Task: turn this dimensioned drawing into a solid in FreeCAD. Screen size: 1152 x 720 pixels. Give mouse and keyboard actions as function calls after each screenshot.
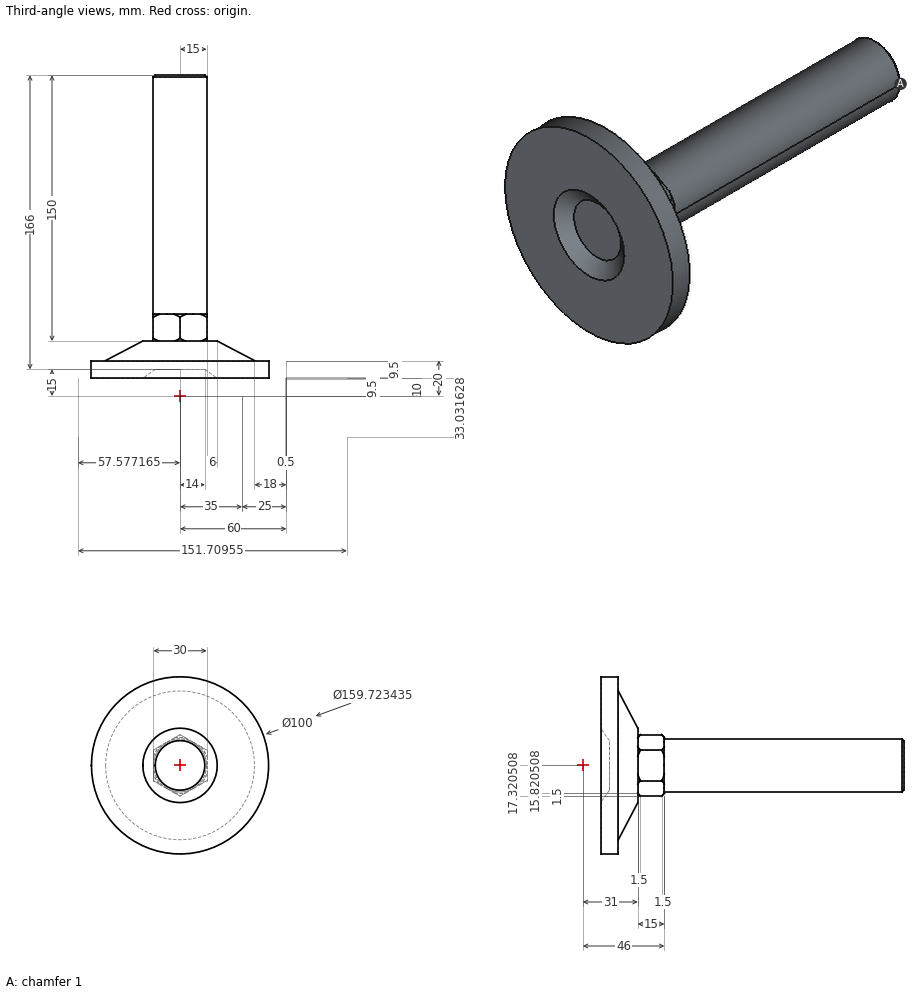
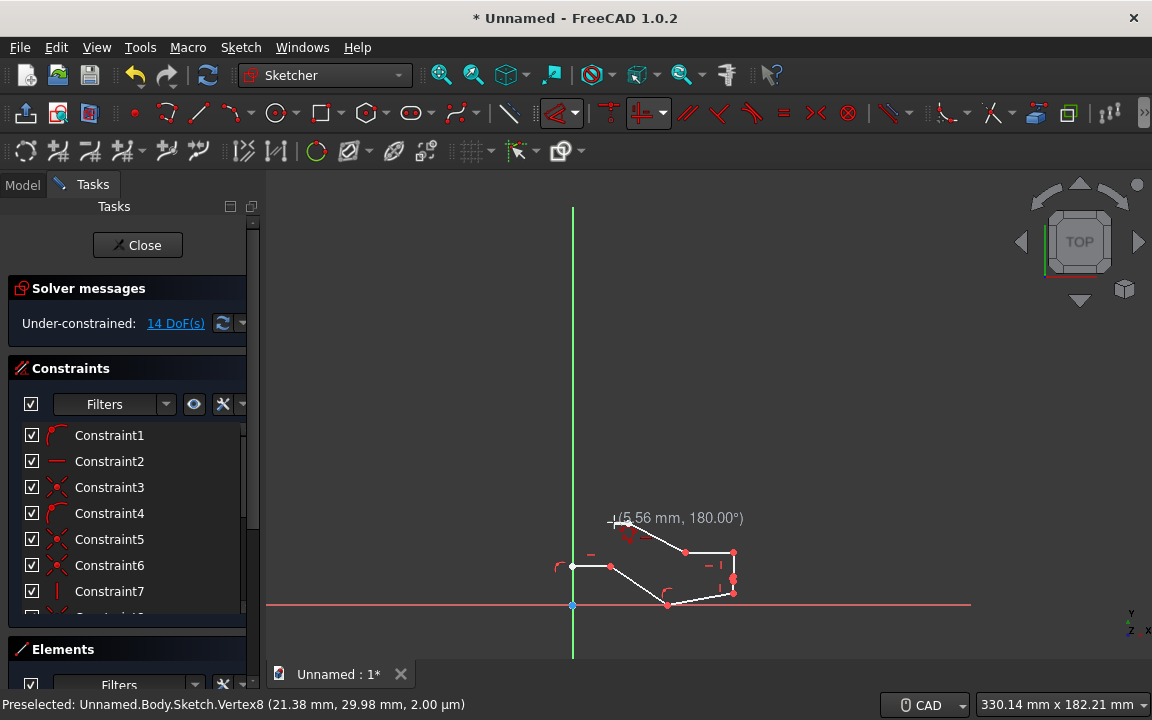
click(613, 522)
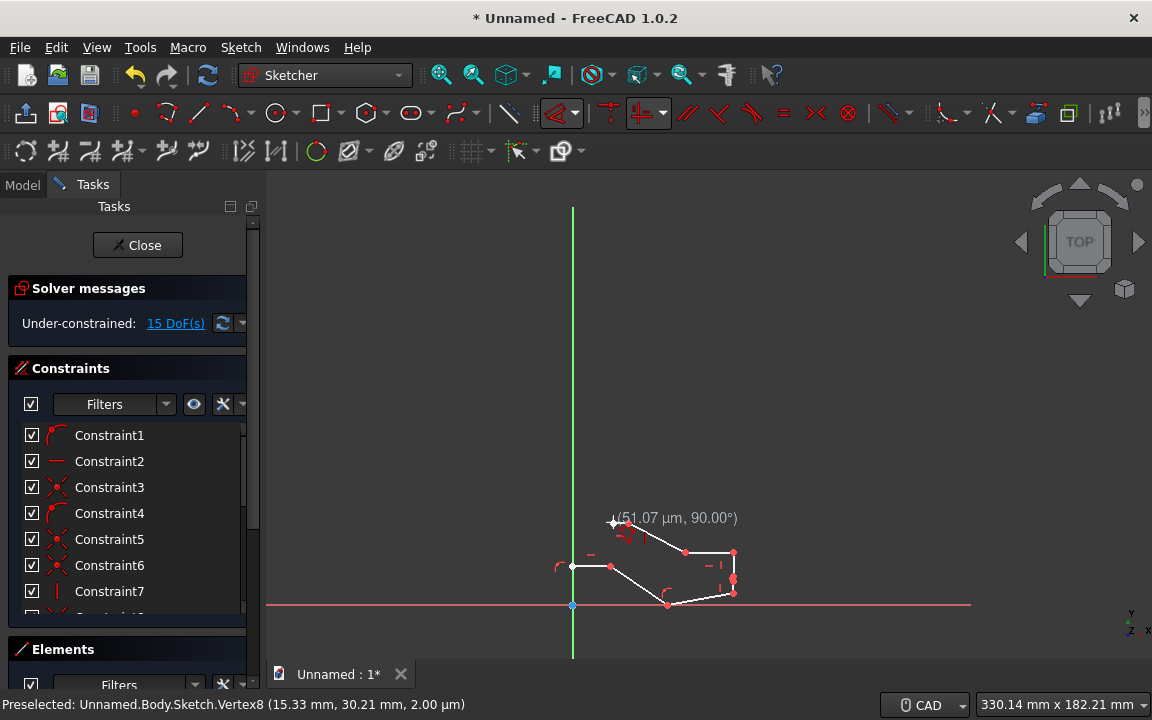
scroll(614, 521, down, 2)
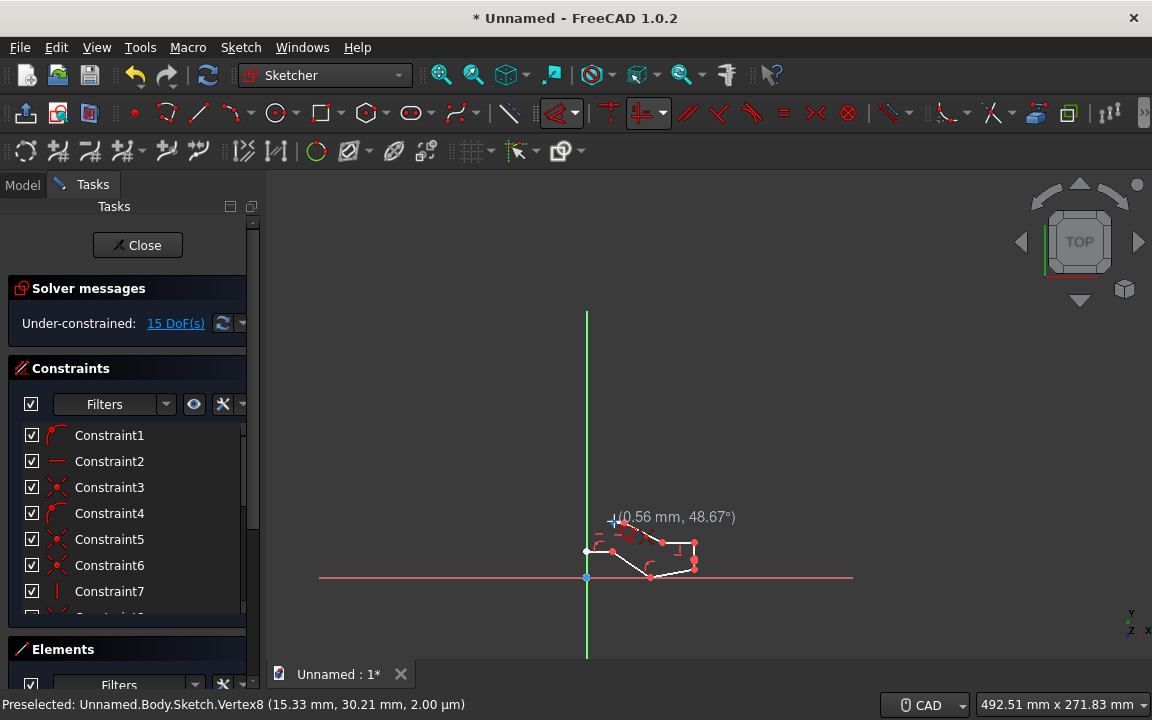
click(613, 252)
click(596, 252)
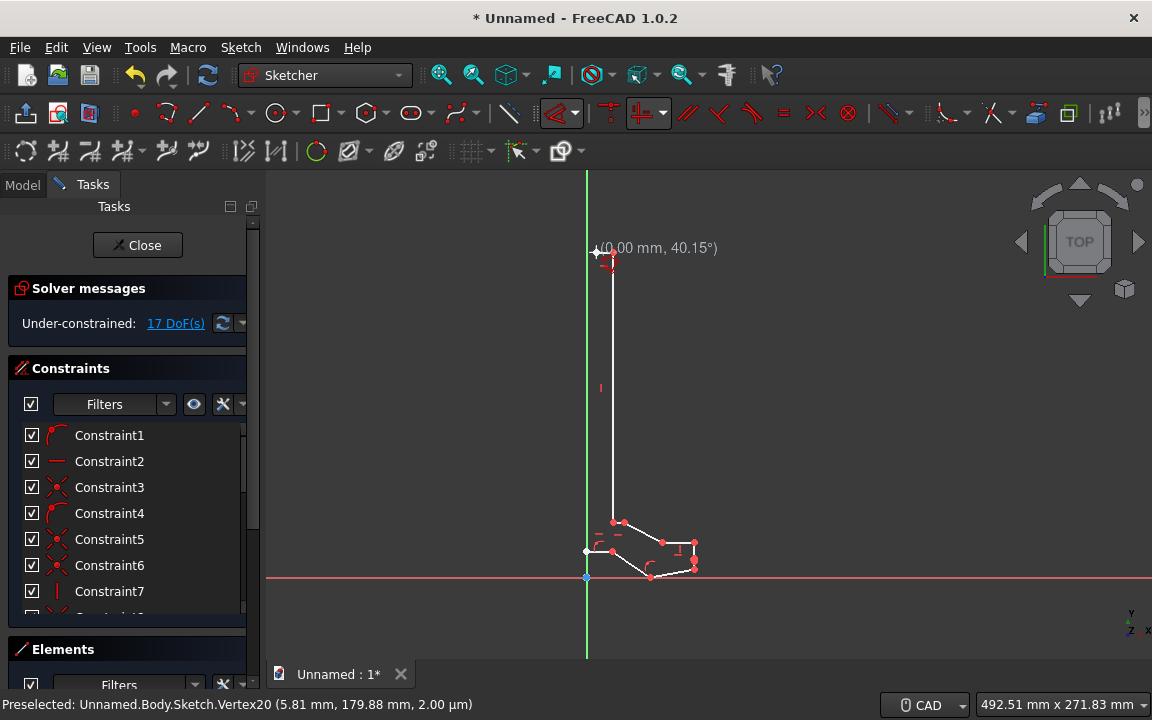
scroll(587, 551, up, 2)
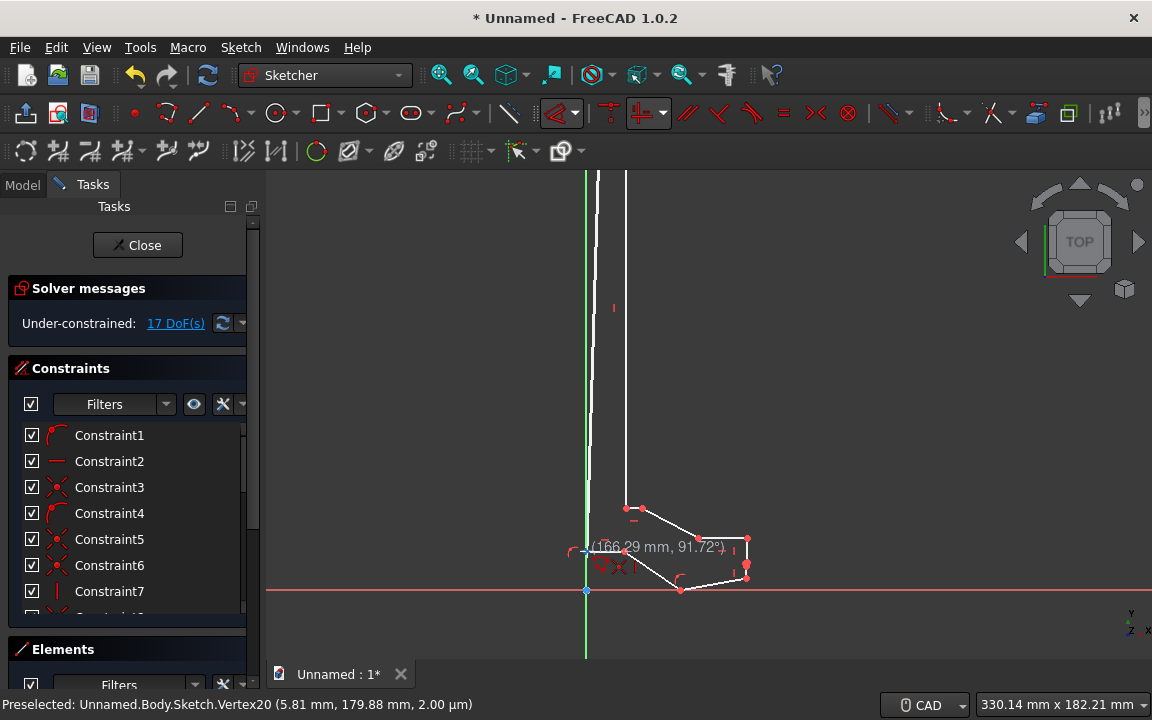
click(586, 552)
key(Escape)
key(Escape)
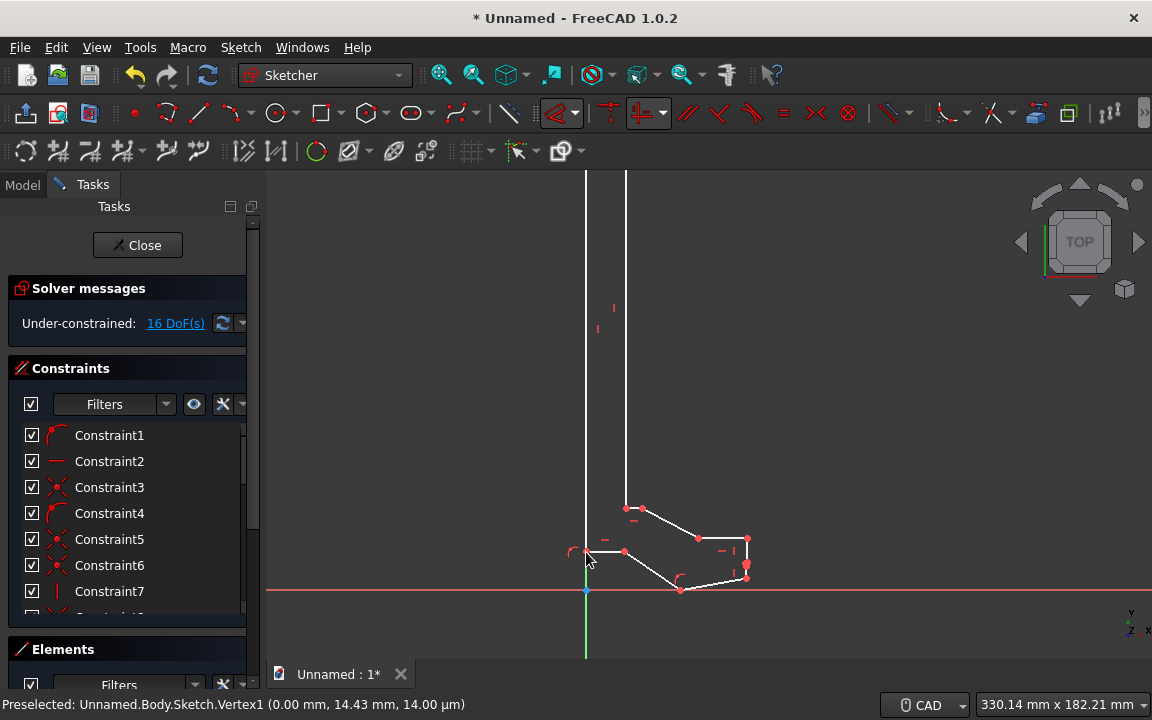
click(700, 587)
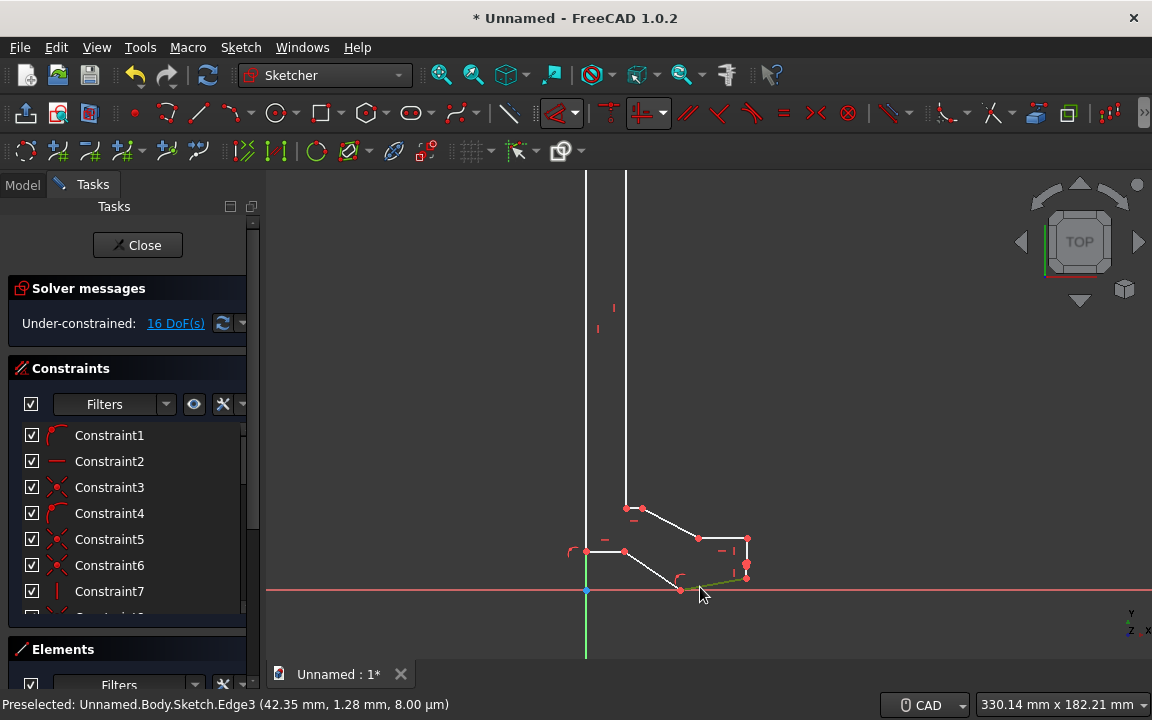
click(666, 114)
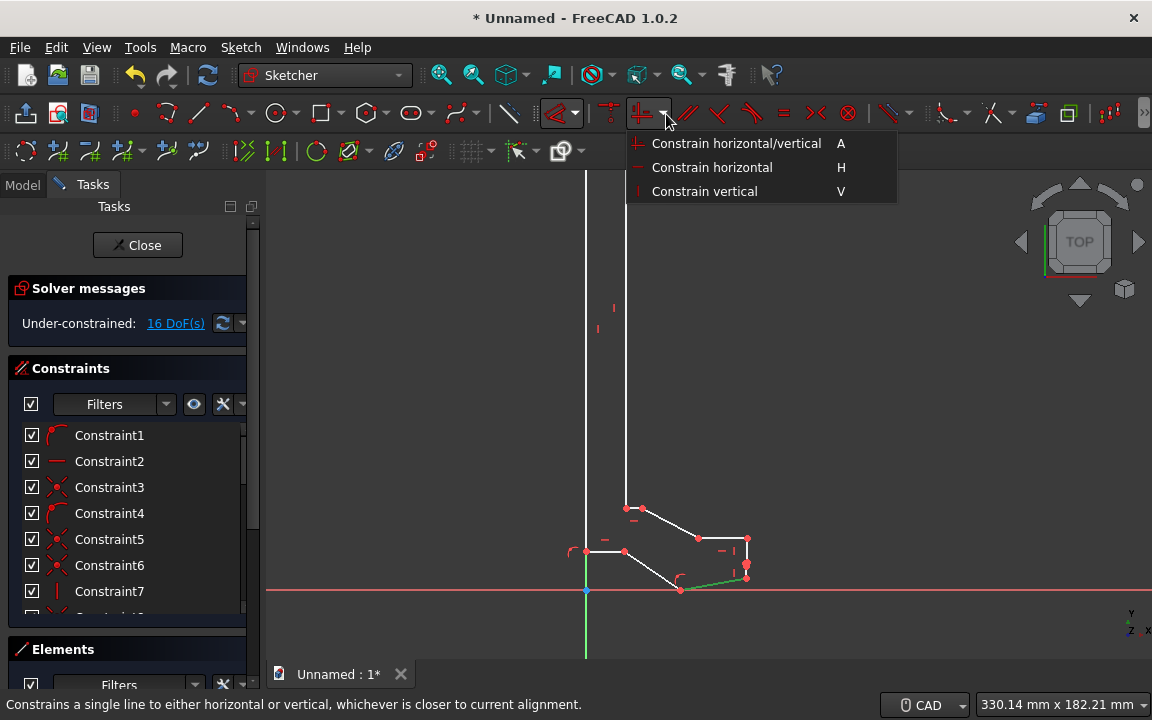
click(762, 167)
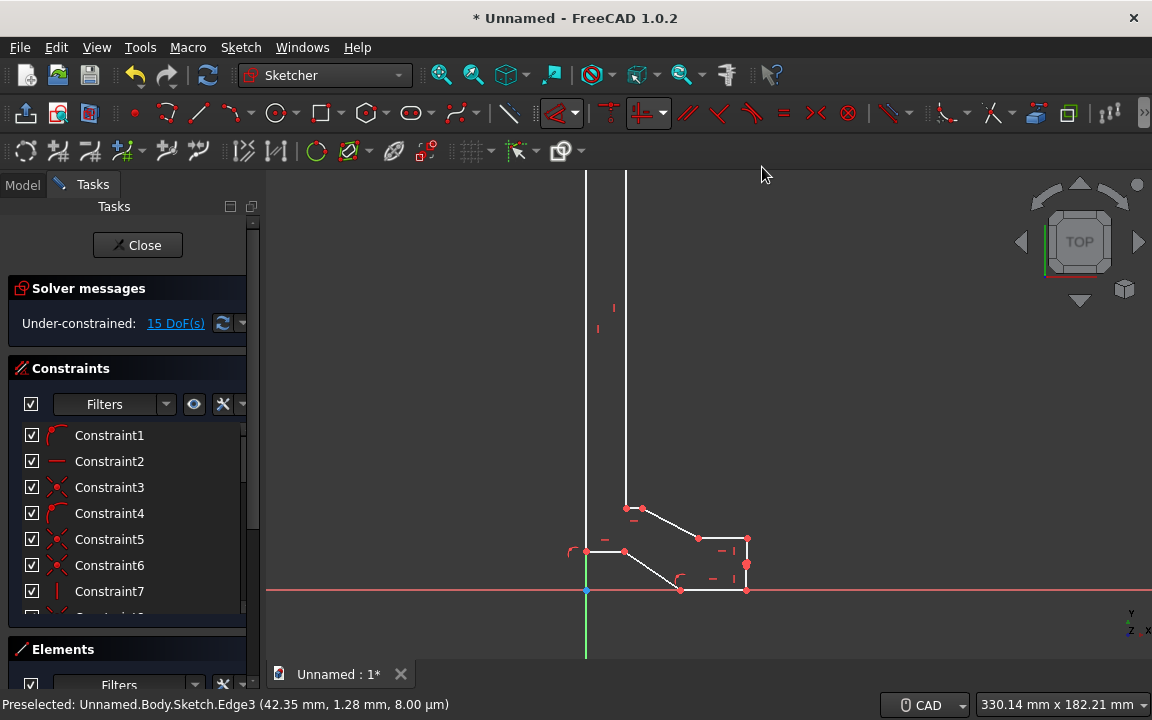
click(556, 114)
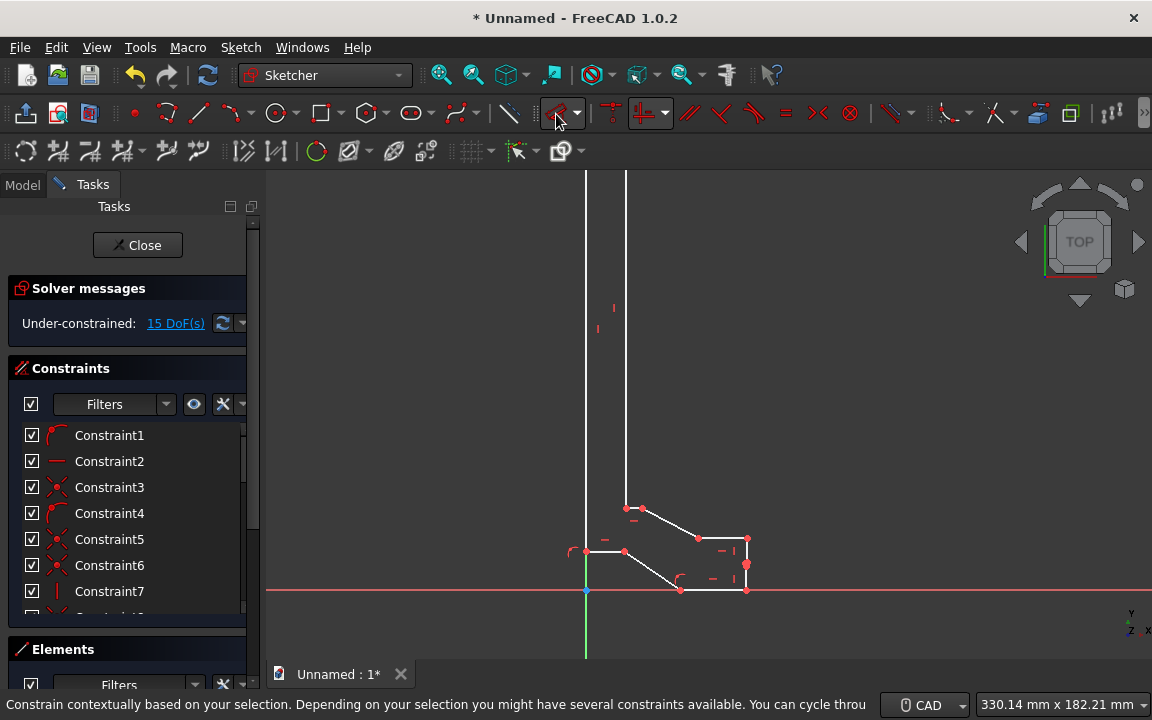
scroll(634, 508, up, 5)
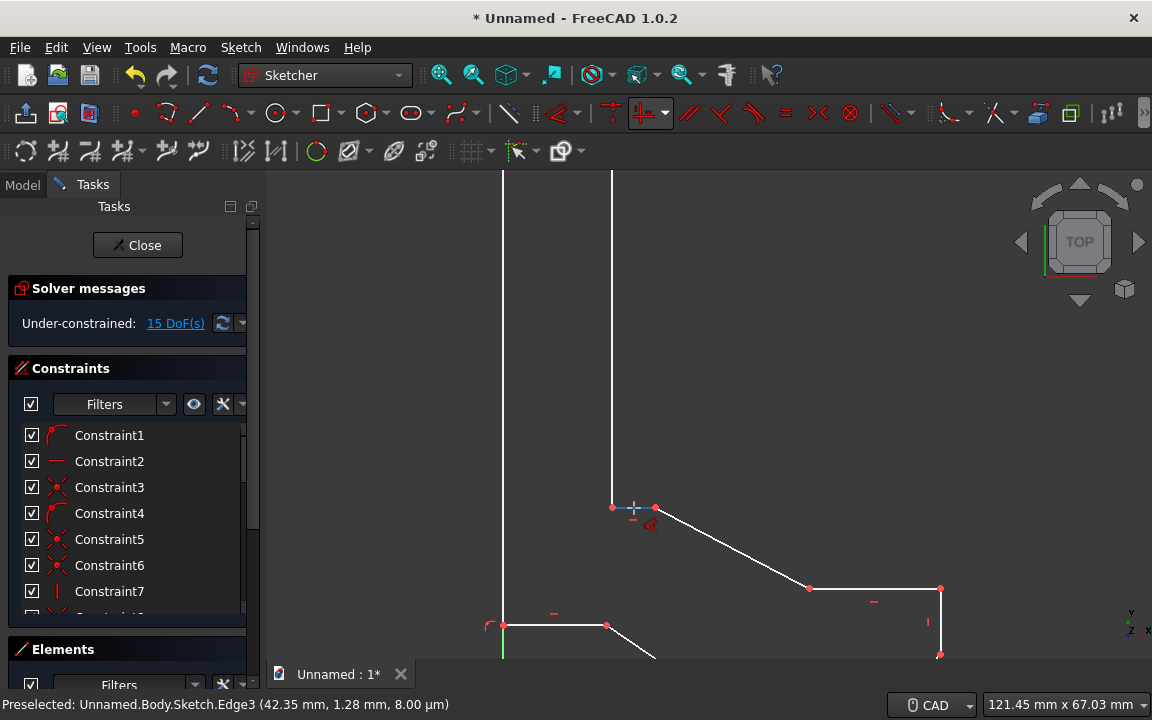
click(634, 508)
click(634, 542)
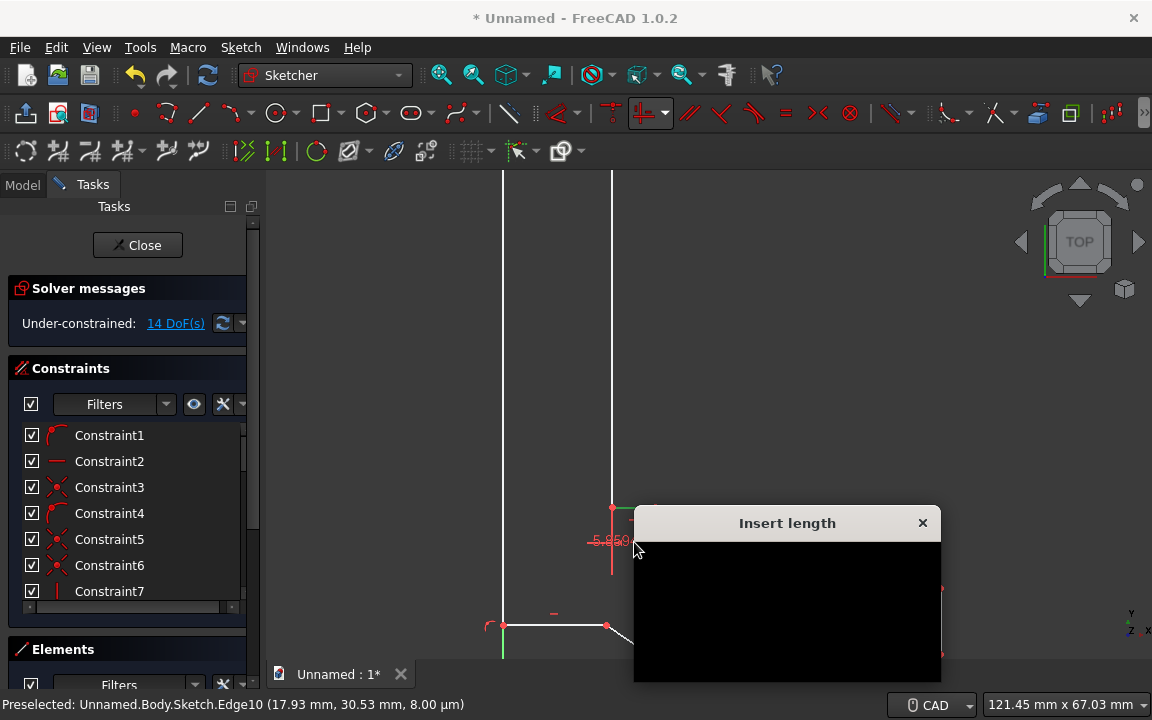
text(6)
key(Return)